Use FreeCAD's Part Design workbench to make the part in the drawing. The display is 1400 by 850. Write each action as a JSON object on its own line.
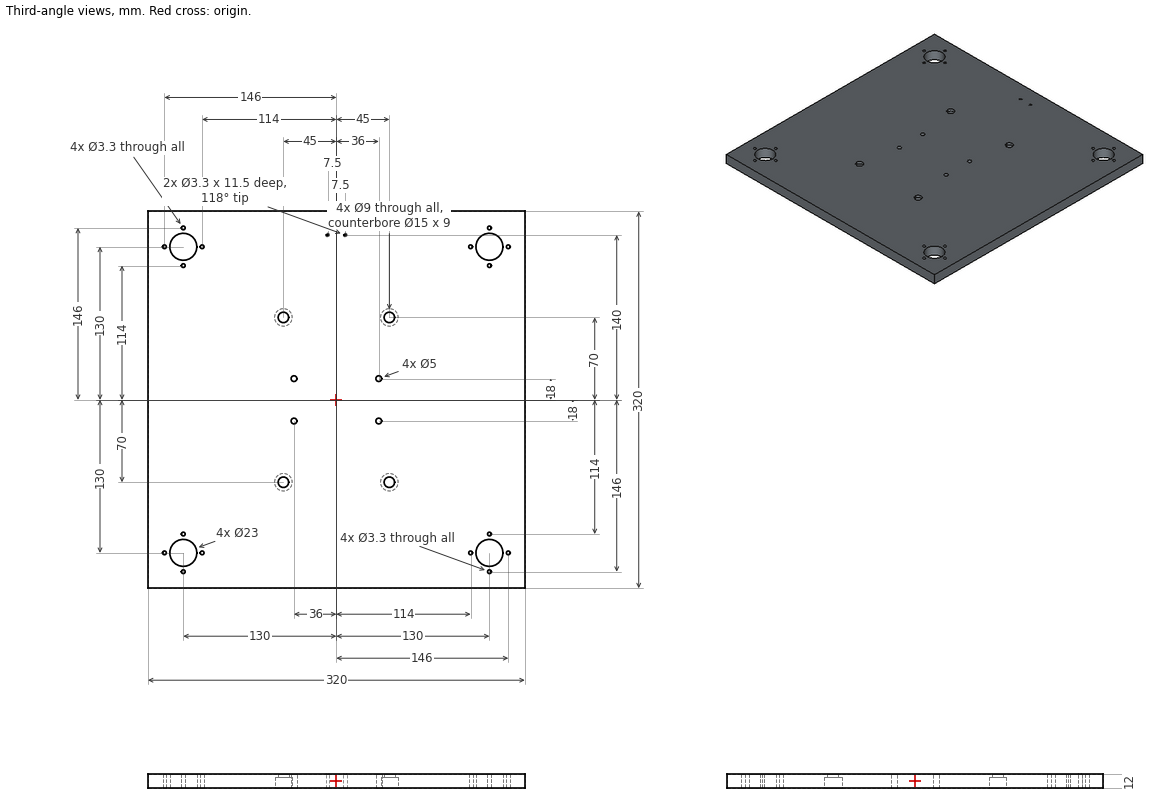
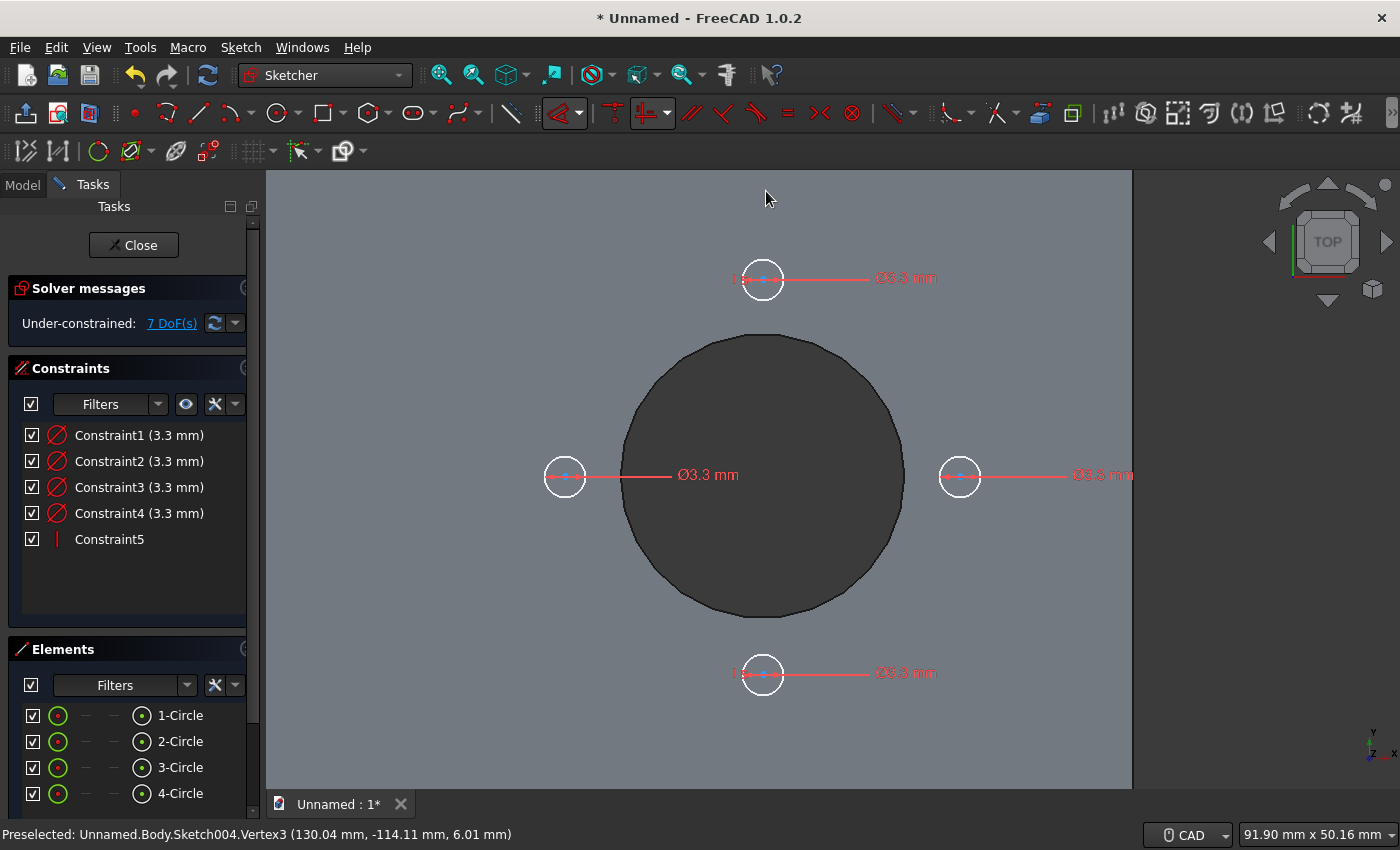
{"action": "left_click", "coordinate": [565, 477]}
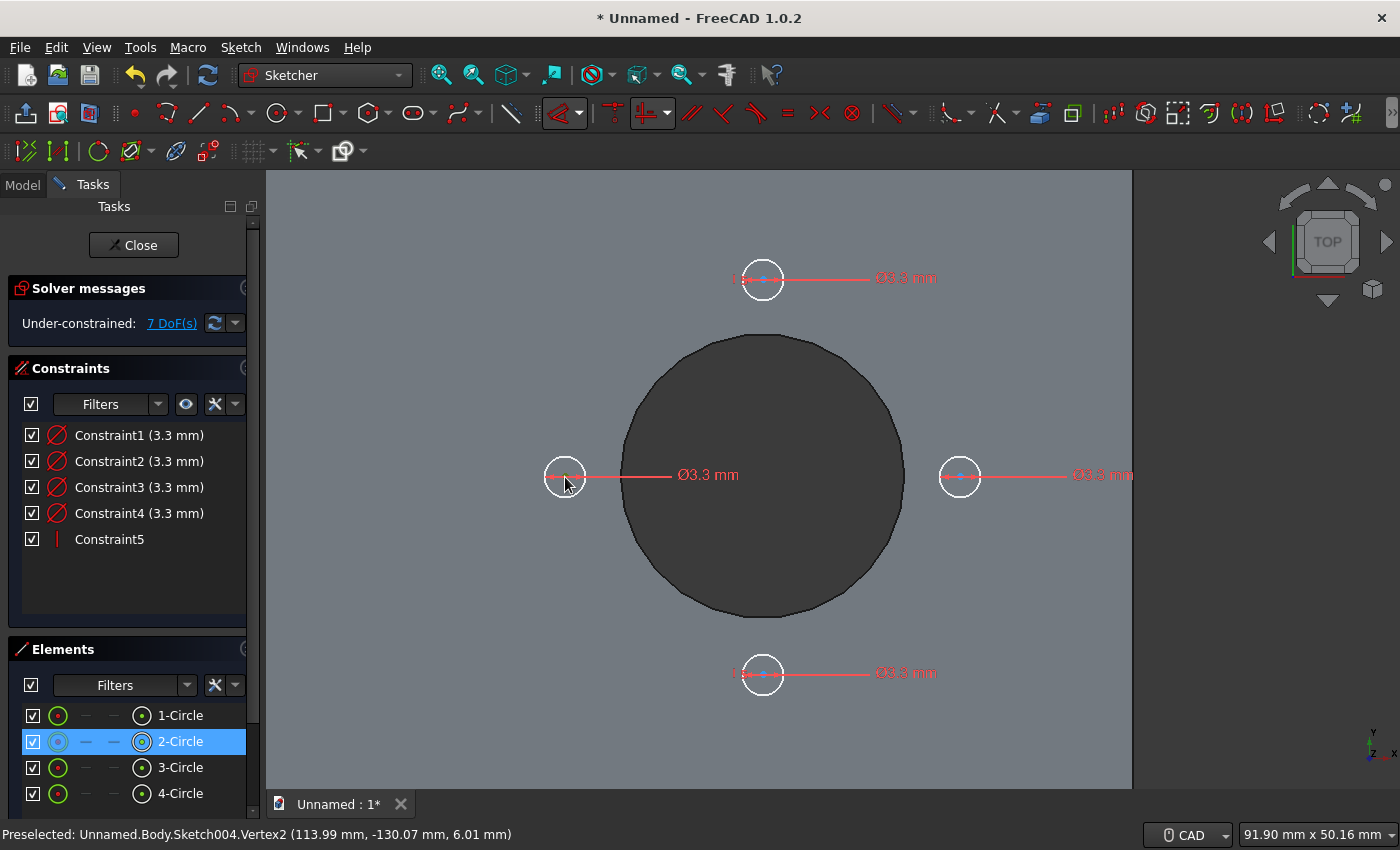
{"action": "left_click", "coordinate": [960, 477]}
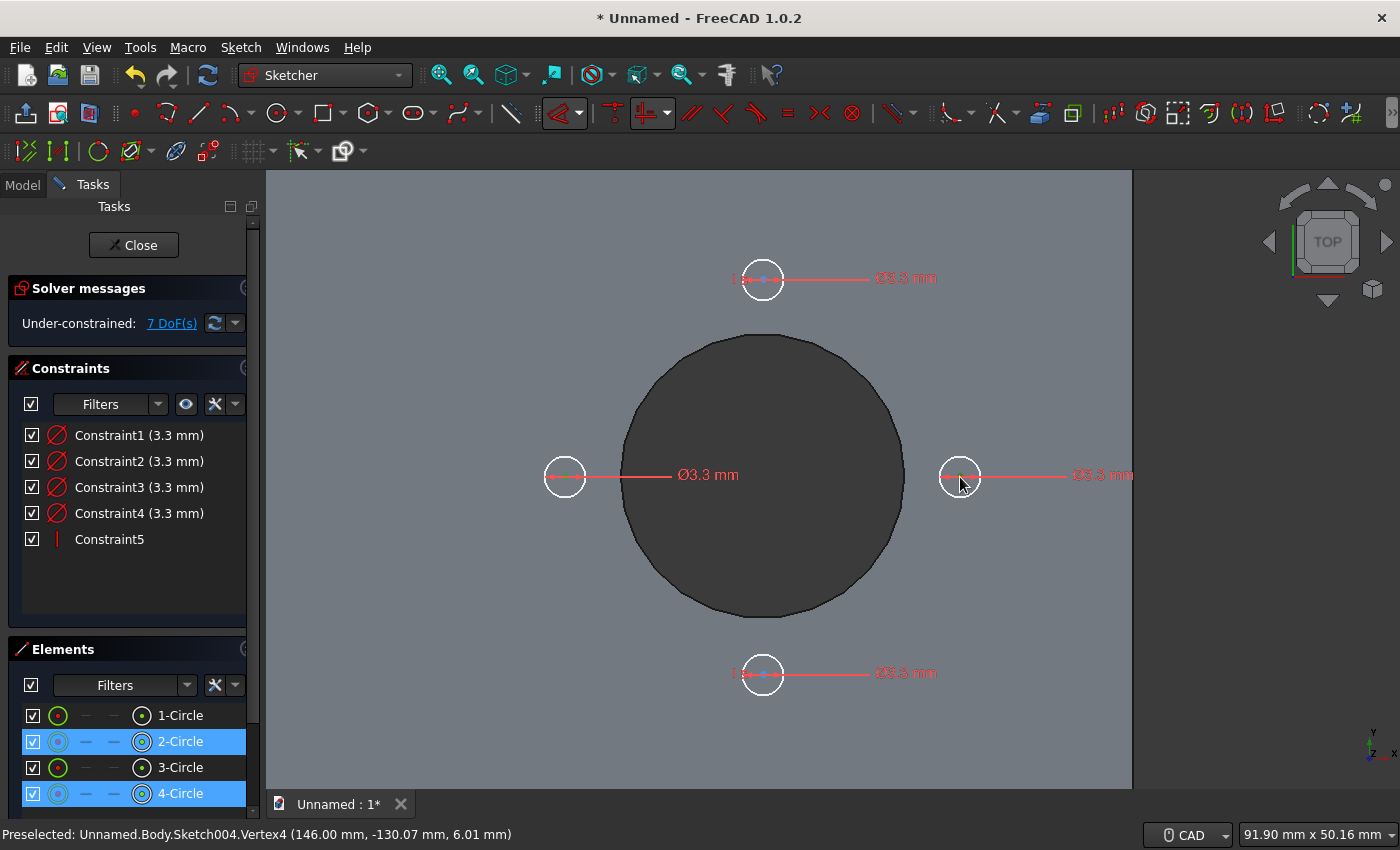
{"action": "left_click", "coordinate": [670, 114]}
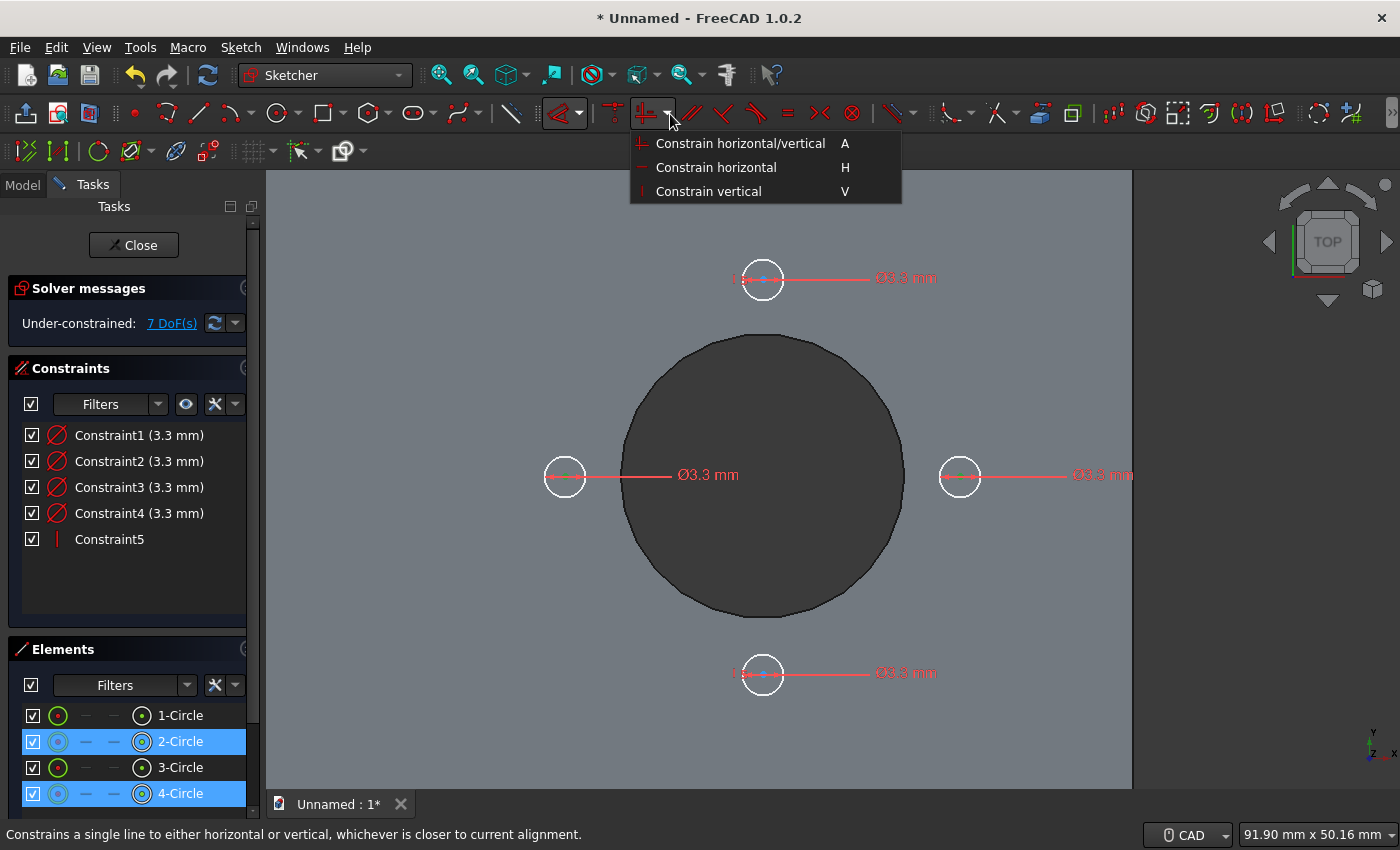
{"action": "left_click", "coordinate": [766, 167]}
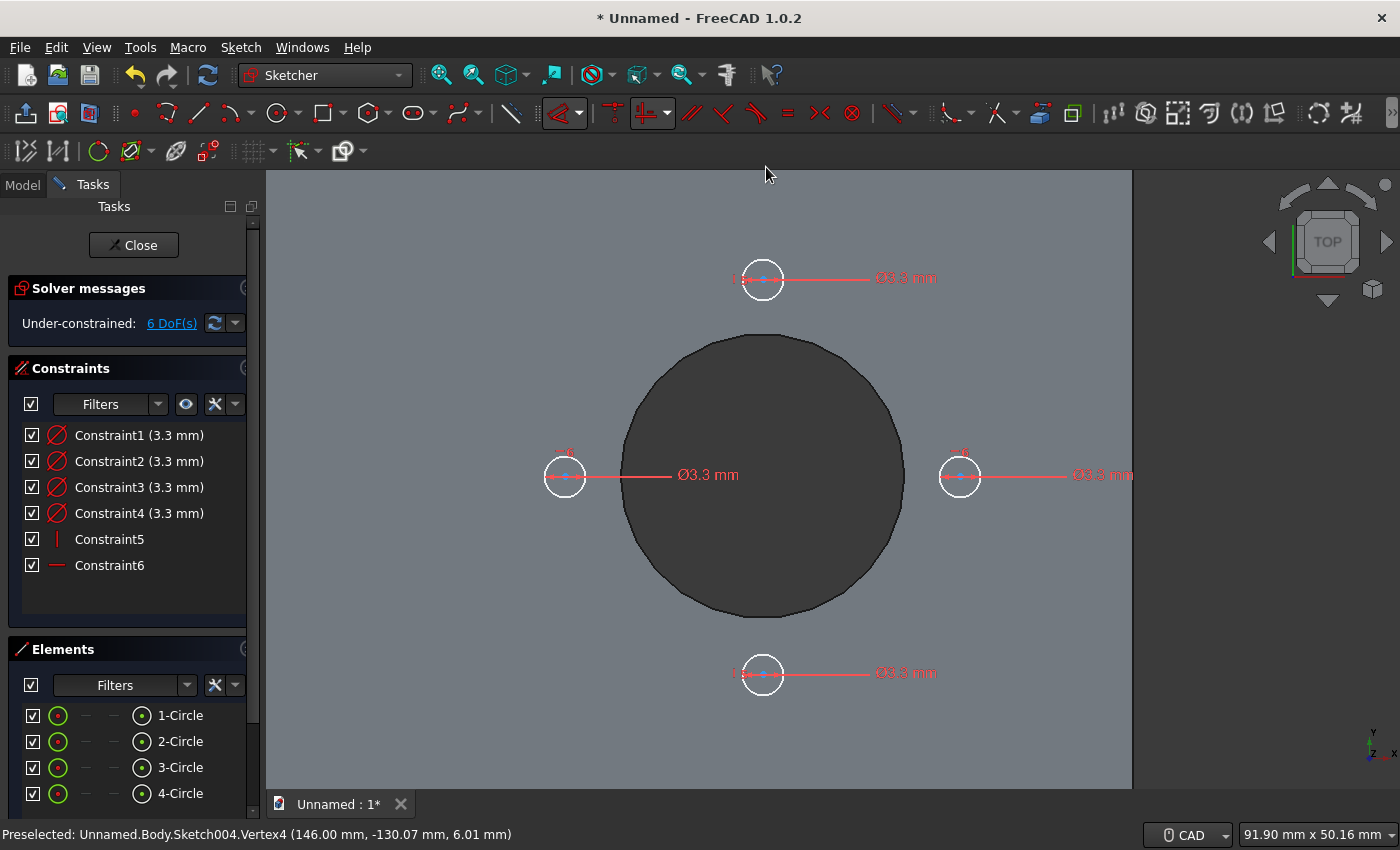
{"action": "left_click", "coordinate": [763, 675]}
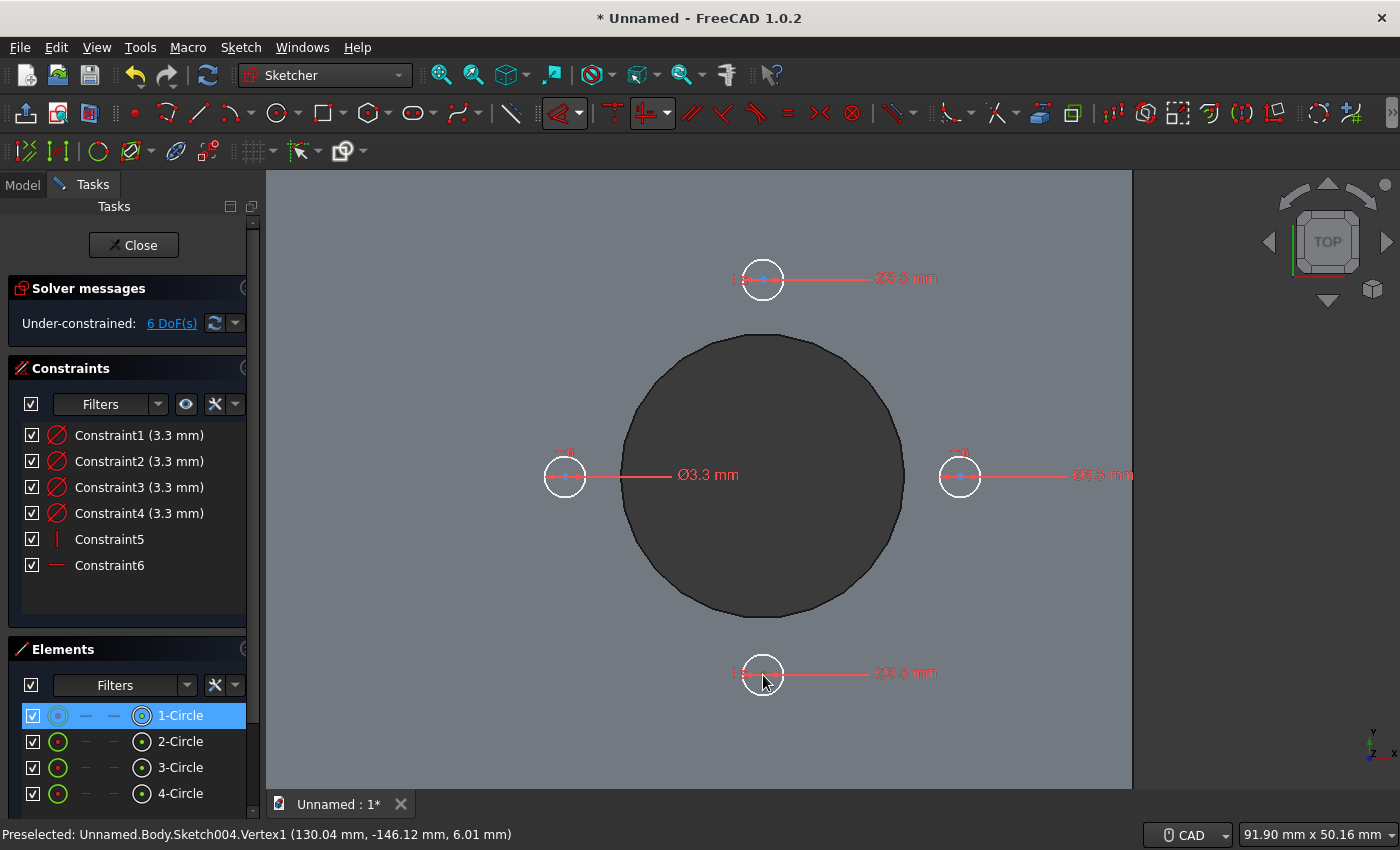
{"action": "left_click", "coordinate": [582, 114]}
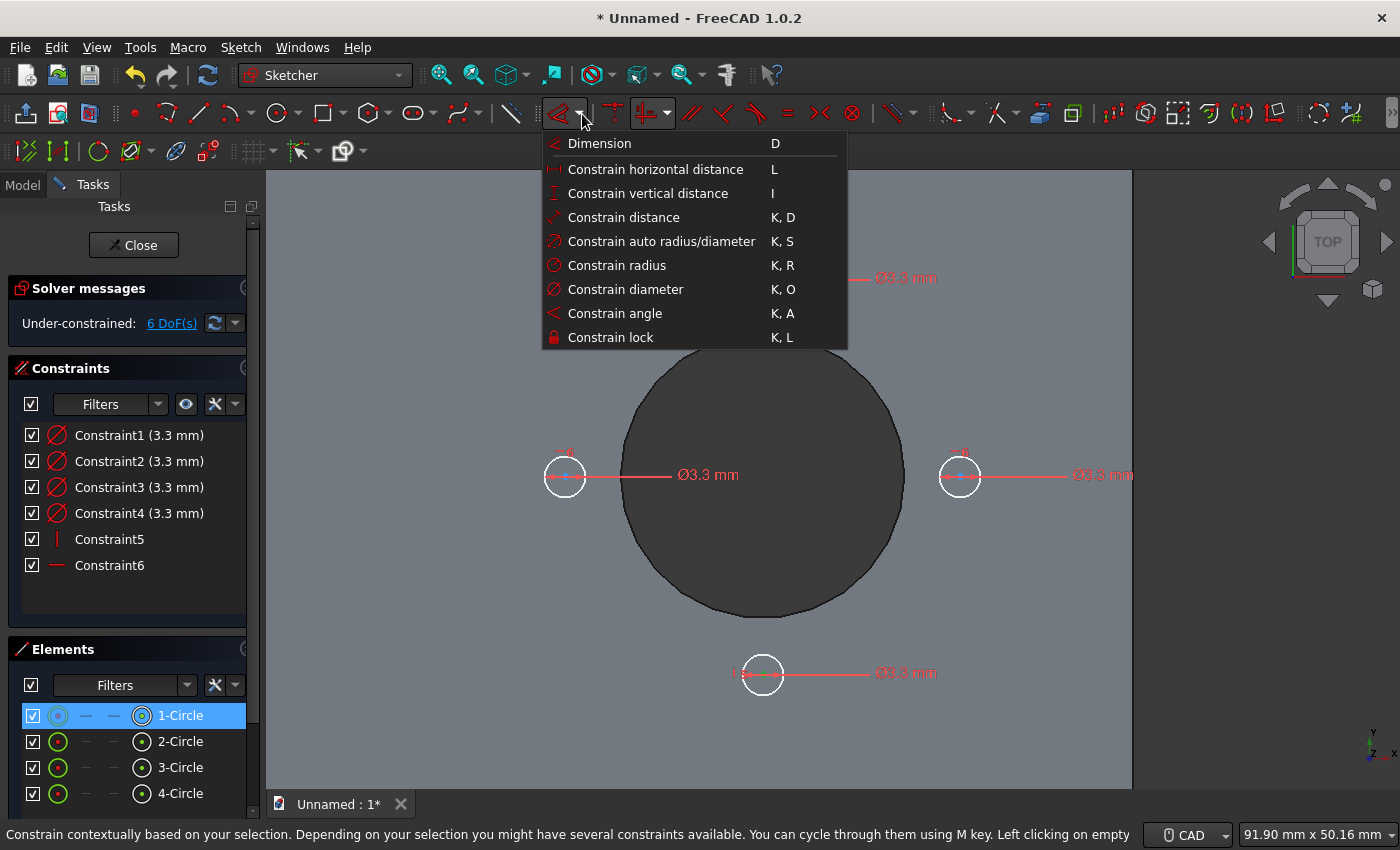
{"action": "left_click", "coordinate": [695, 169]}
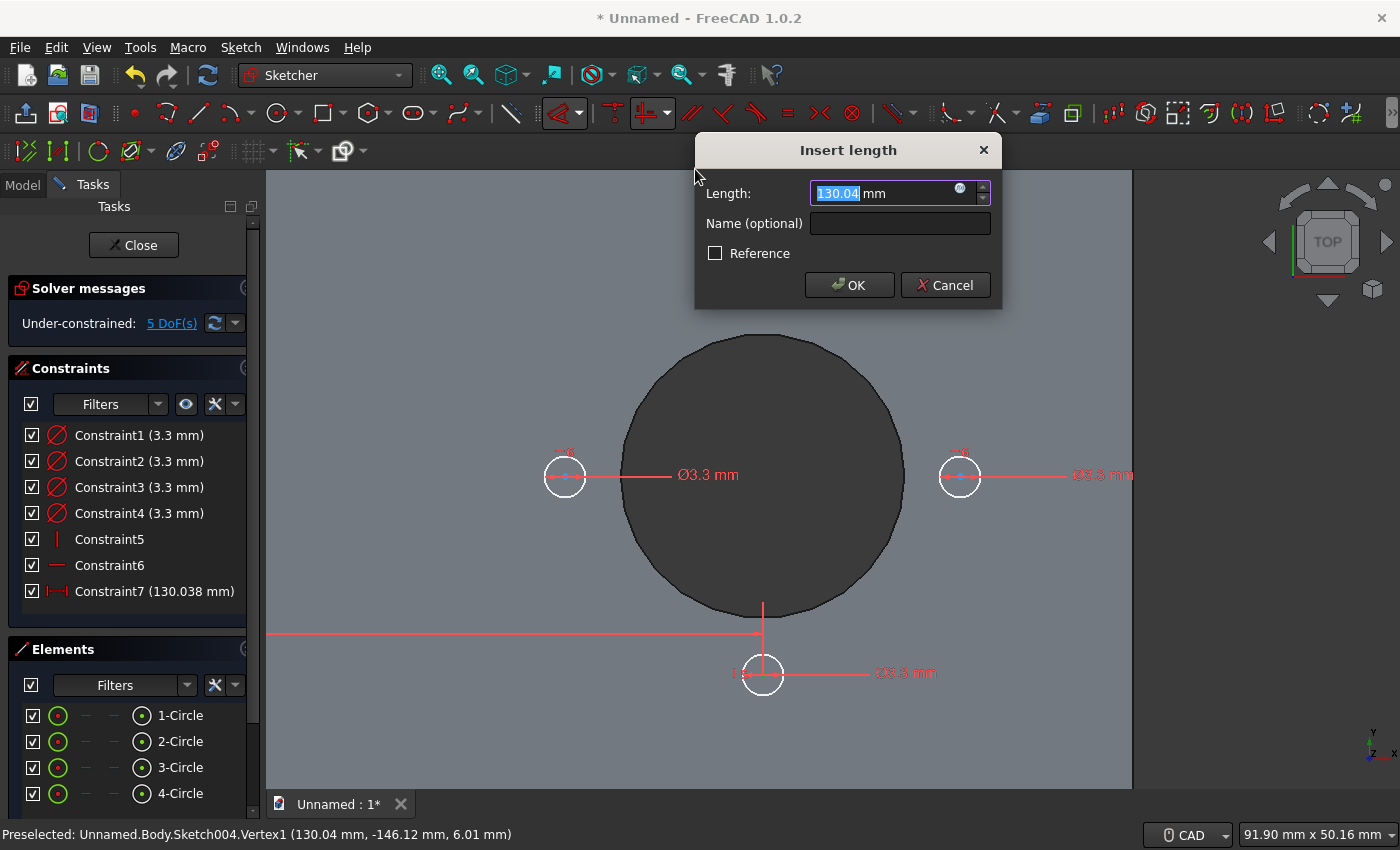
{"action": "type", "text": "130"}
{"action": "key", "text": "Return"}